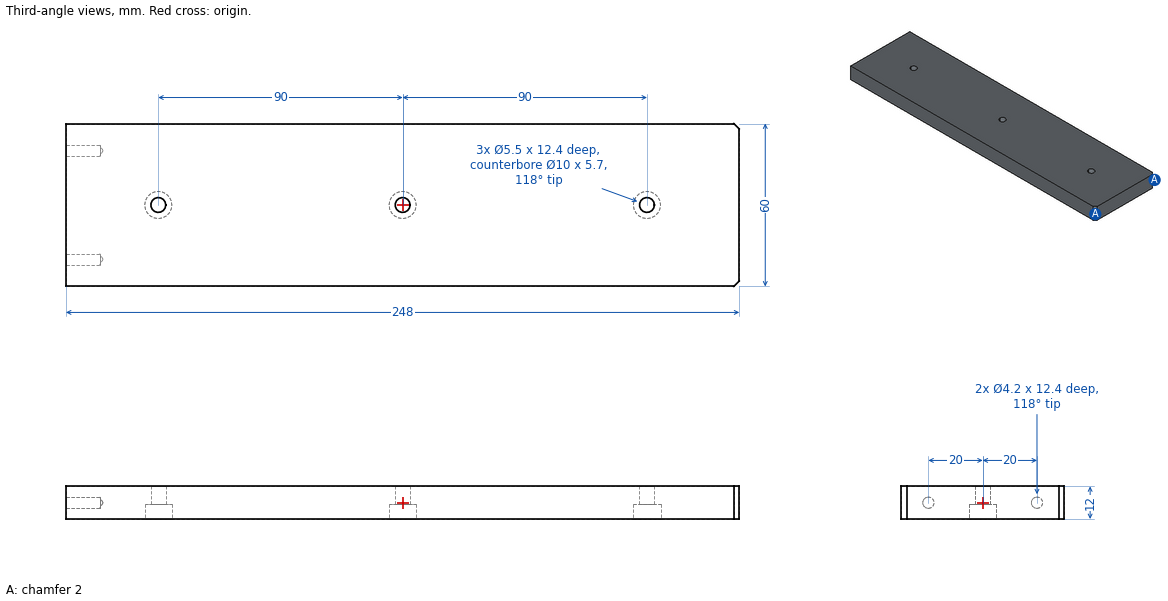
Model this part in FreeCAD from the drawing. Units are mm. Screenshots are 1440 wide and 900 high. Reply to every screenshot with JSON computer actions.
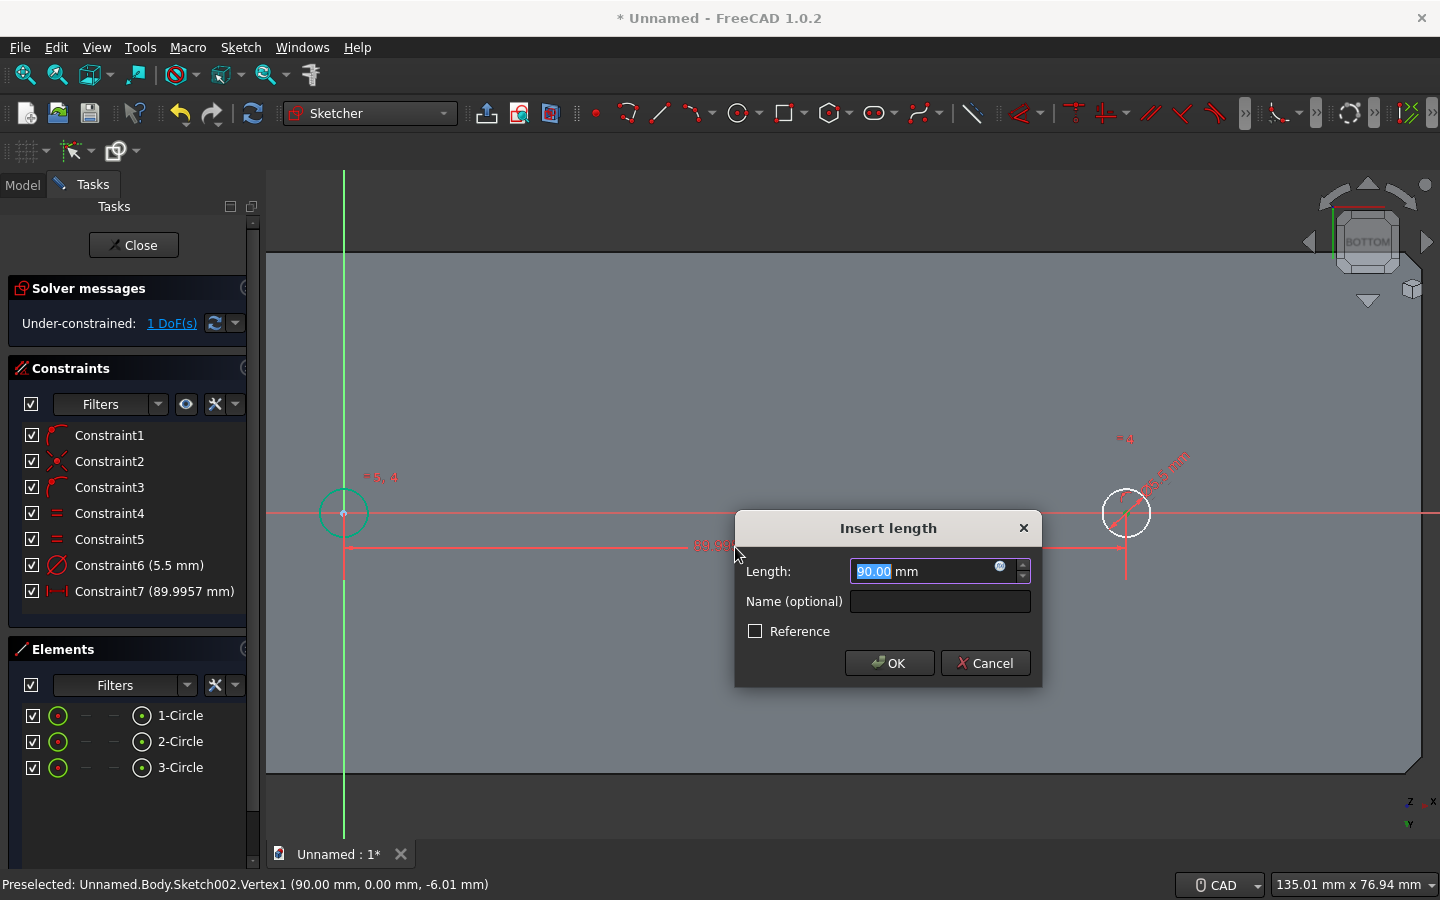
{"action": "type", "text": "90"}
{"action": "key", "text": "Return"}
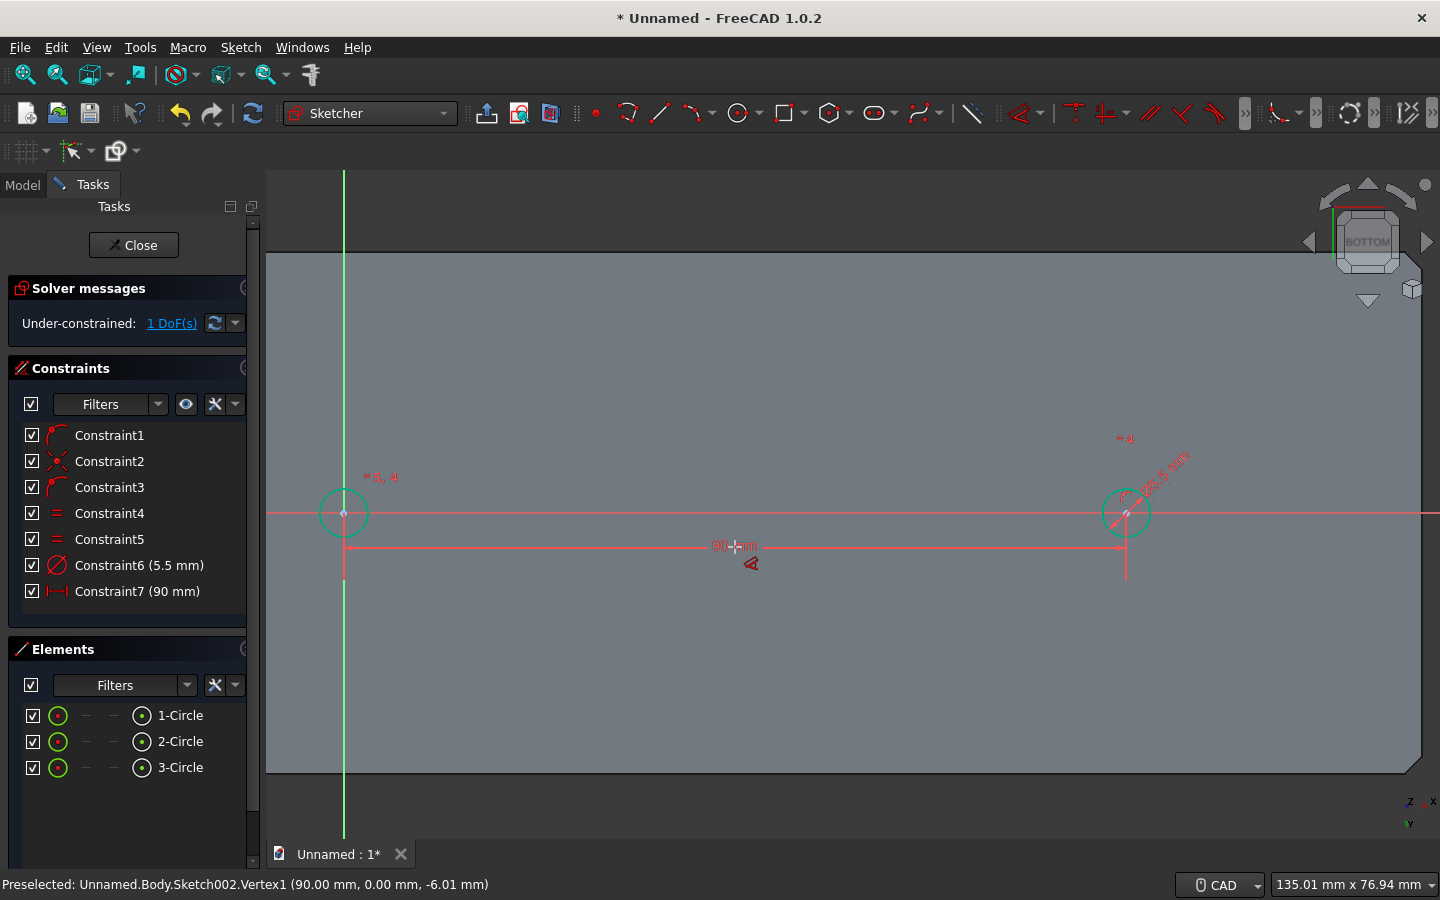
{"action": "scroll", "coordinate": [1144, 497], "scroll_direction": "down", "scroll_amount": 4}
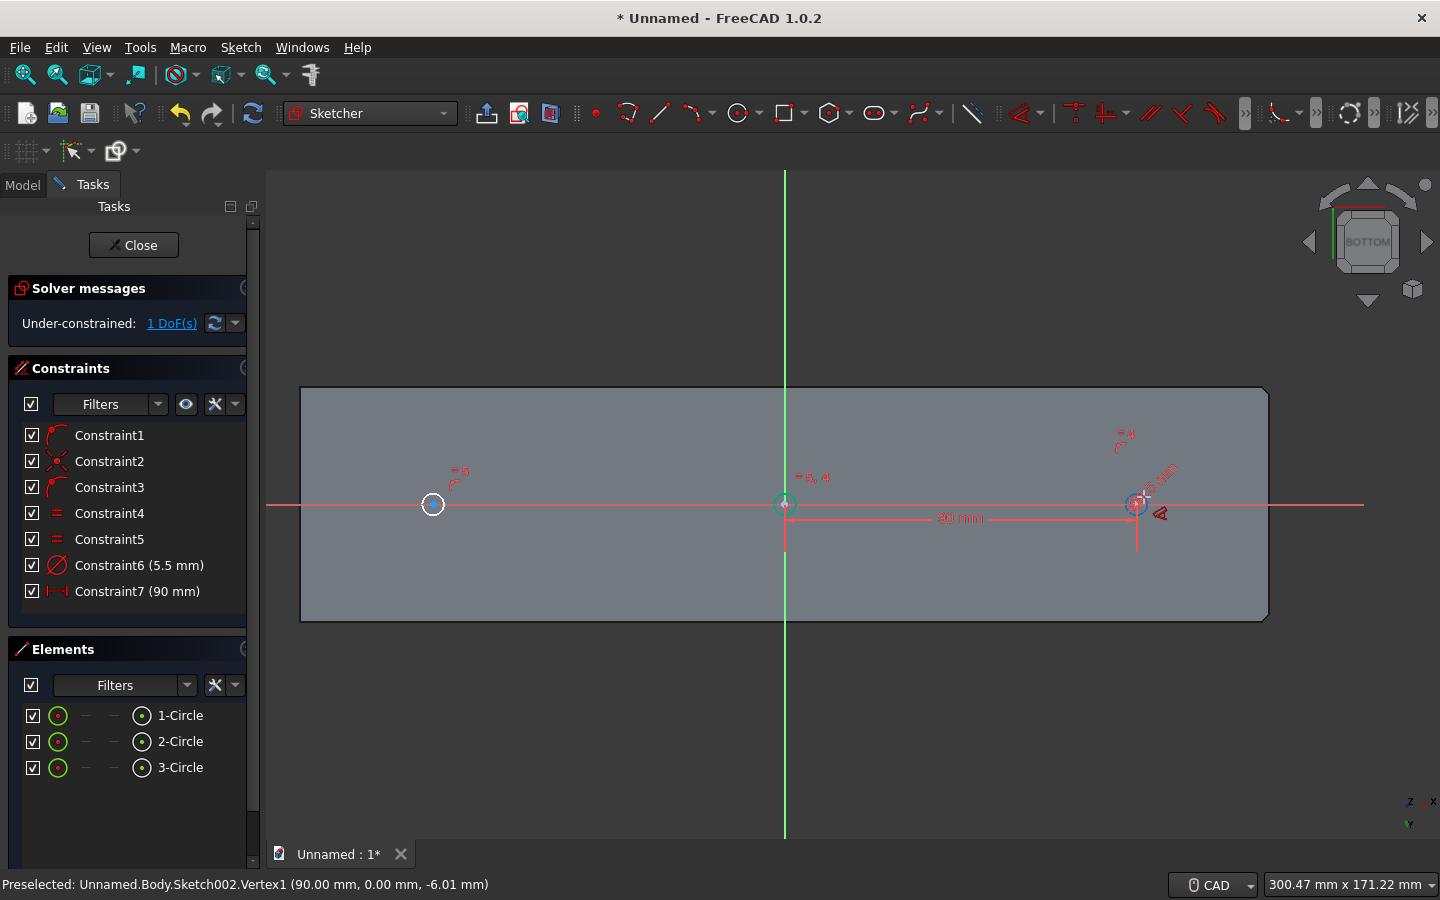
{"action": "left_click", "coordinate": [433, 505]}
{"action": "left_click", "coordinate": [609, 539]}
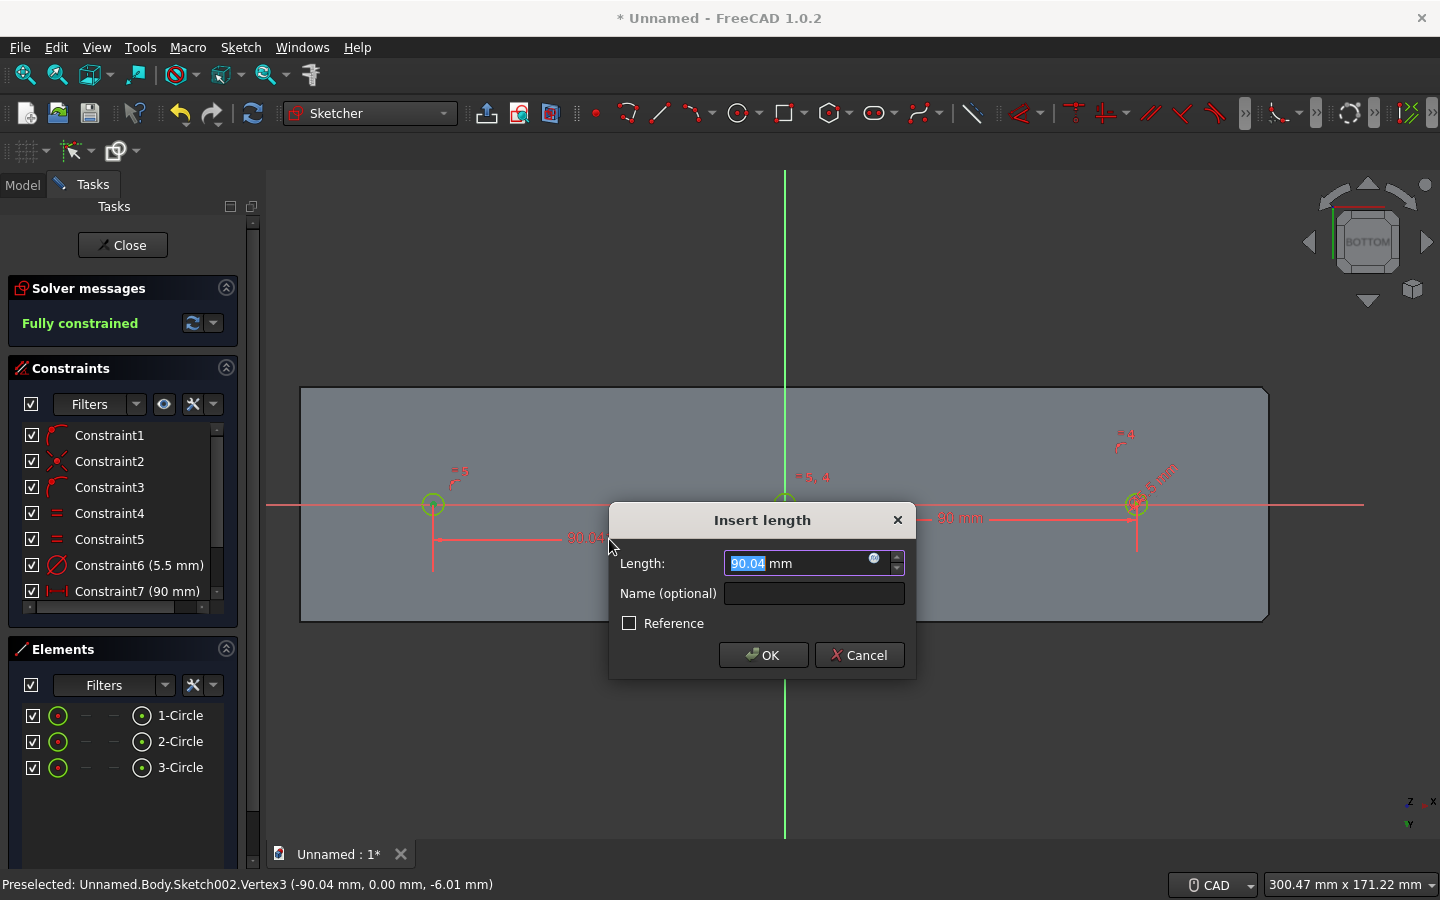
{"action": "type", "text": "90"}
{"action": "key", "text": "Return"}
{"action": "key", "text": "Escape"}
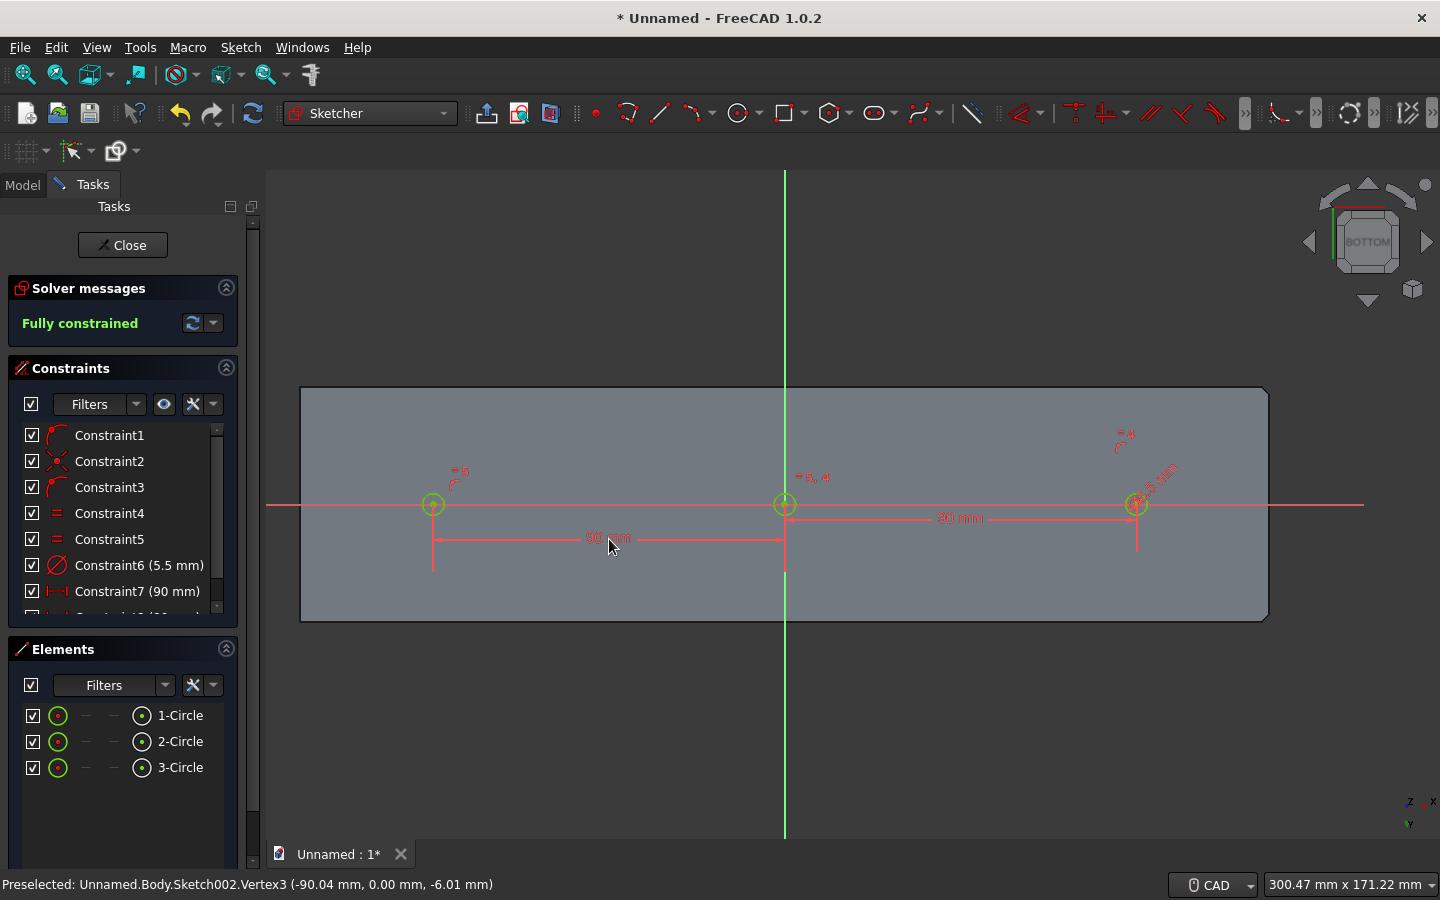
{"action": "left_click", "coordinate": [123, 245]}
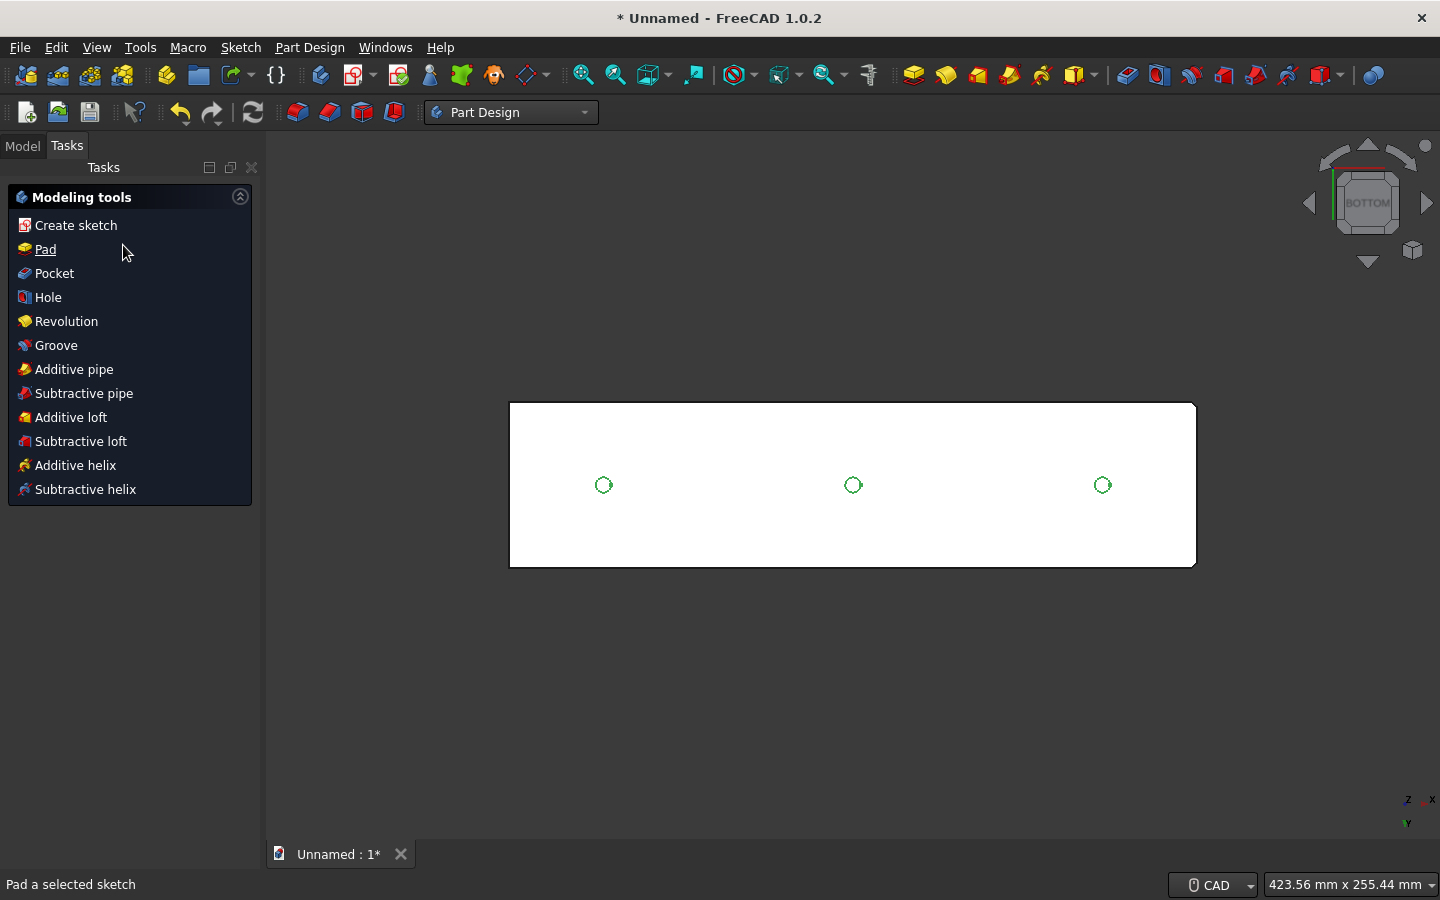
{"action": "left_click", "coordinate": [1160, 76]}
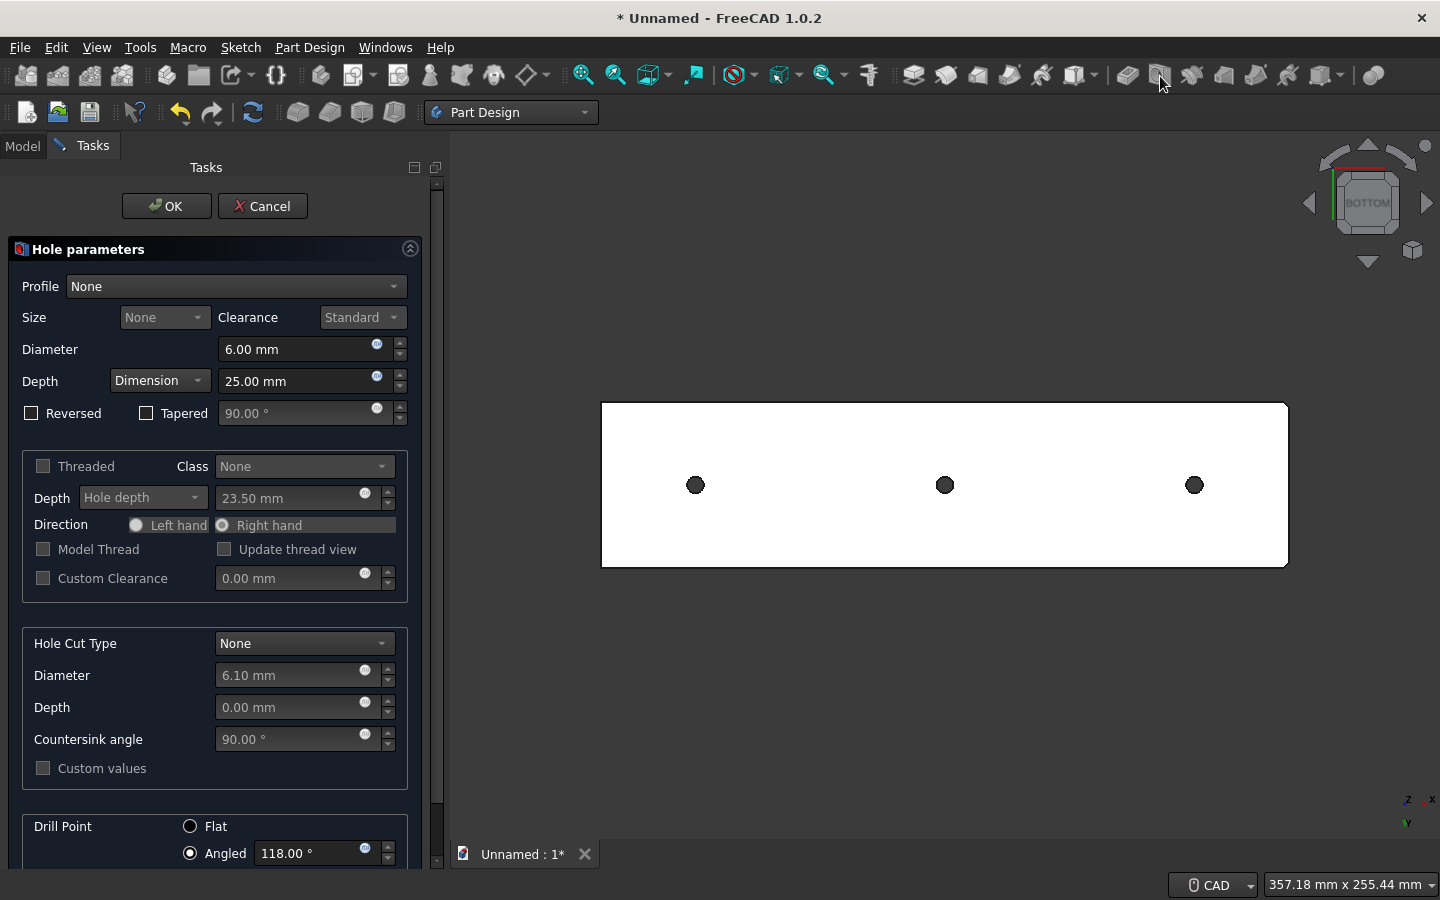
{"action": "triple_click", "coordinate": [305, 349]}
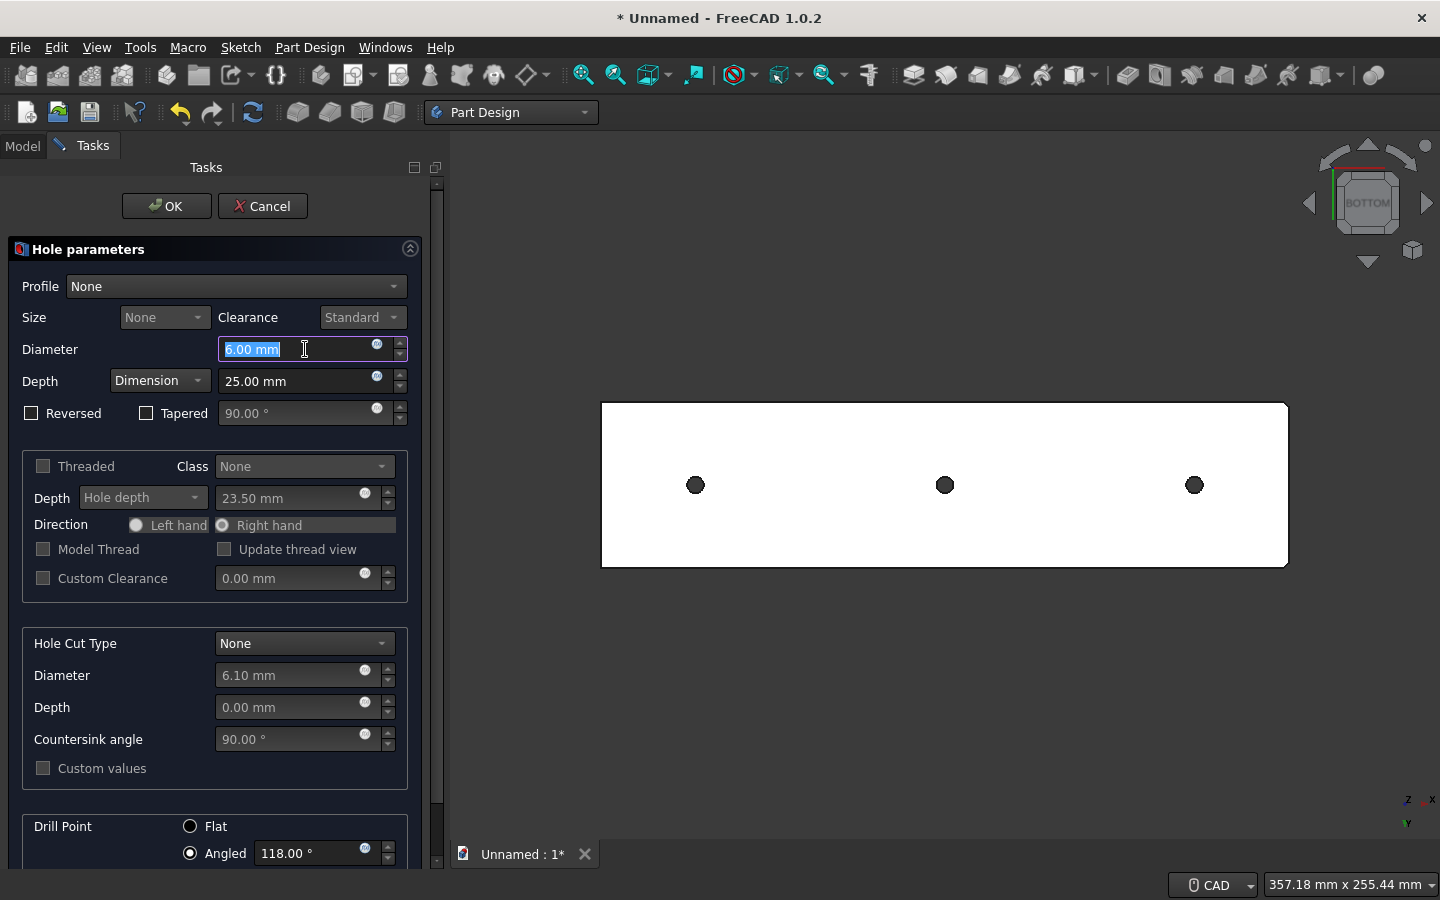
{"action": "type", "text": "5.5"}
{"action": "key", "text": "Tab"}